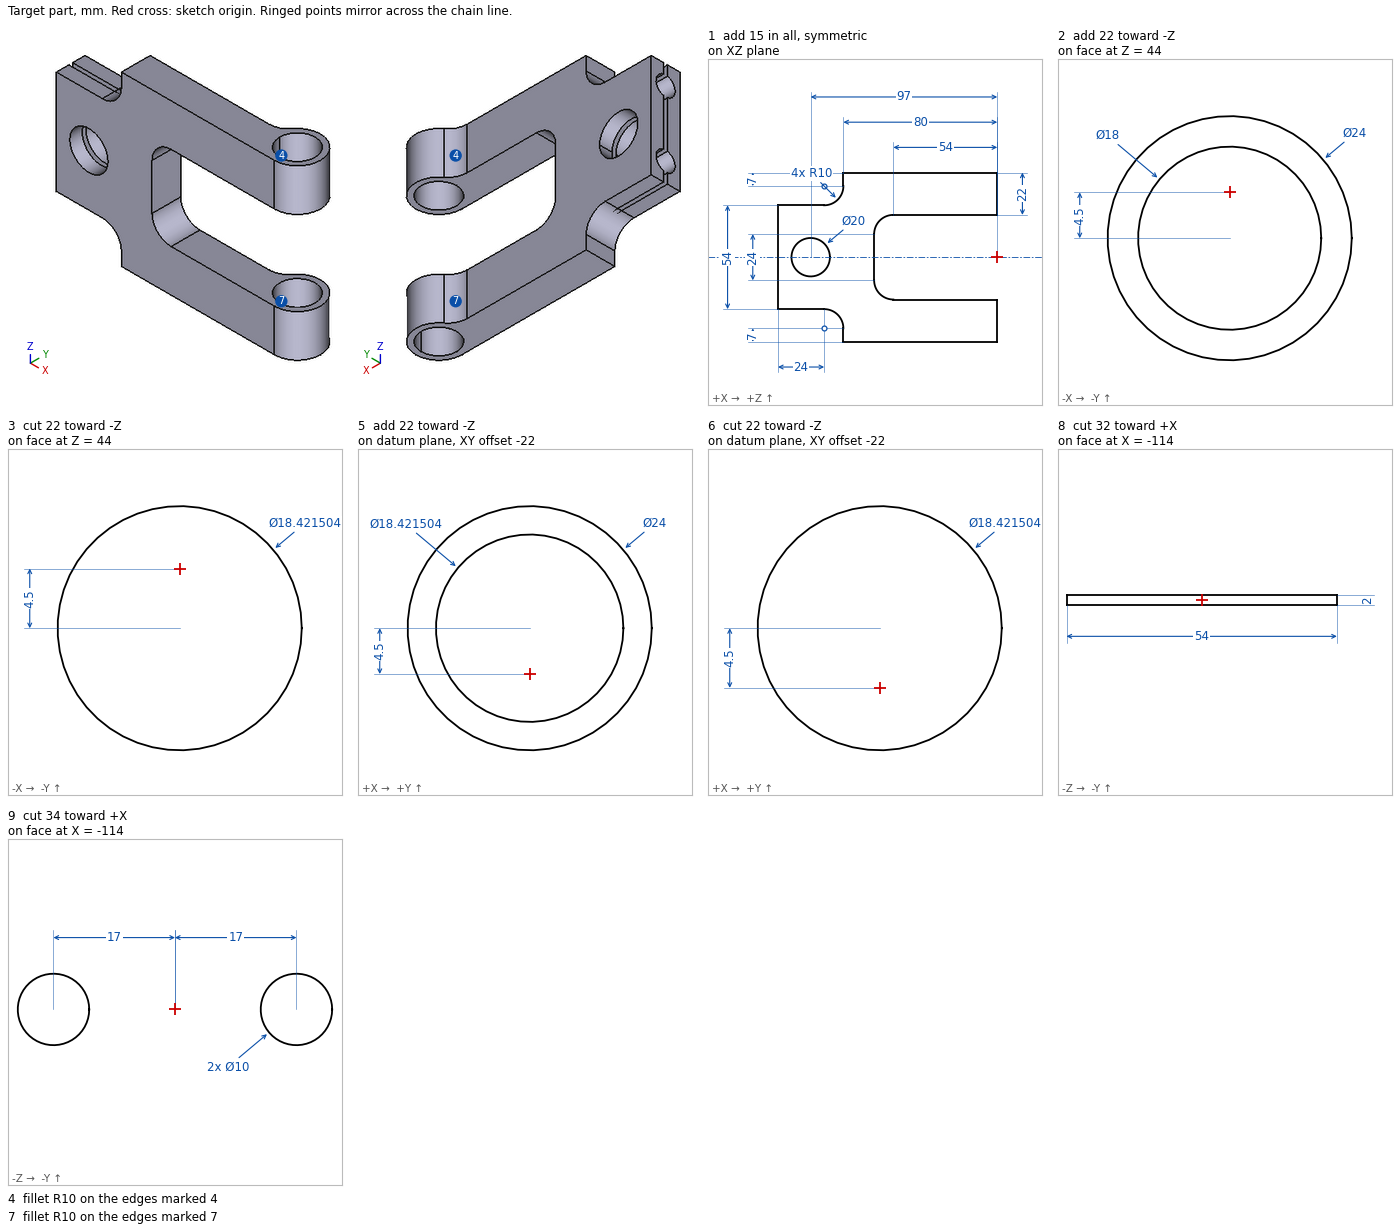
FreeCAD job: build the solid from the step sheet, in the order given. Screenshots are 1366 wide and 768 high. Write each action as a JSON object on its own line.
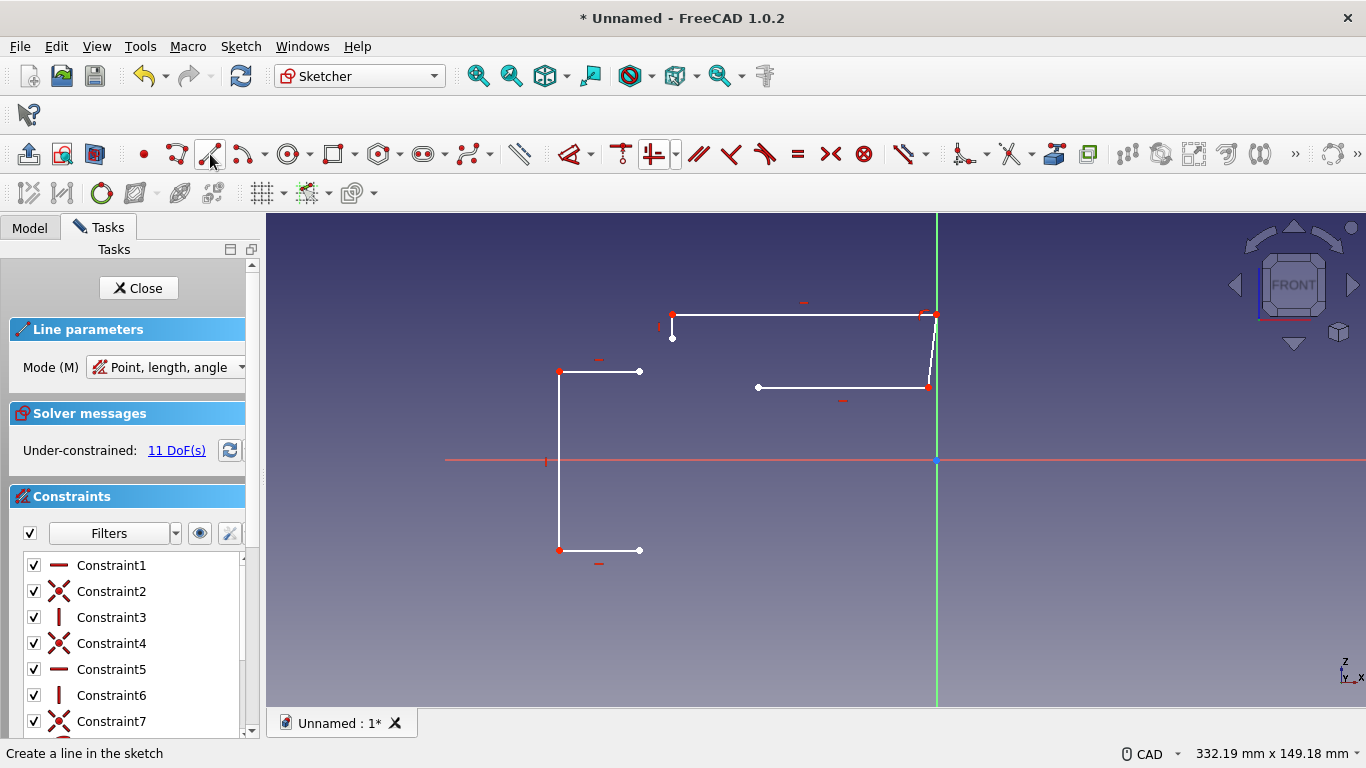
{"action": "left_click", "coordinate": [725, 420]}
{"action": "left_click", "coordinate": [725, 500]}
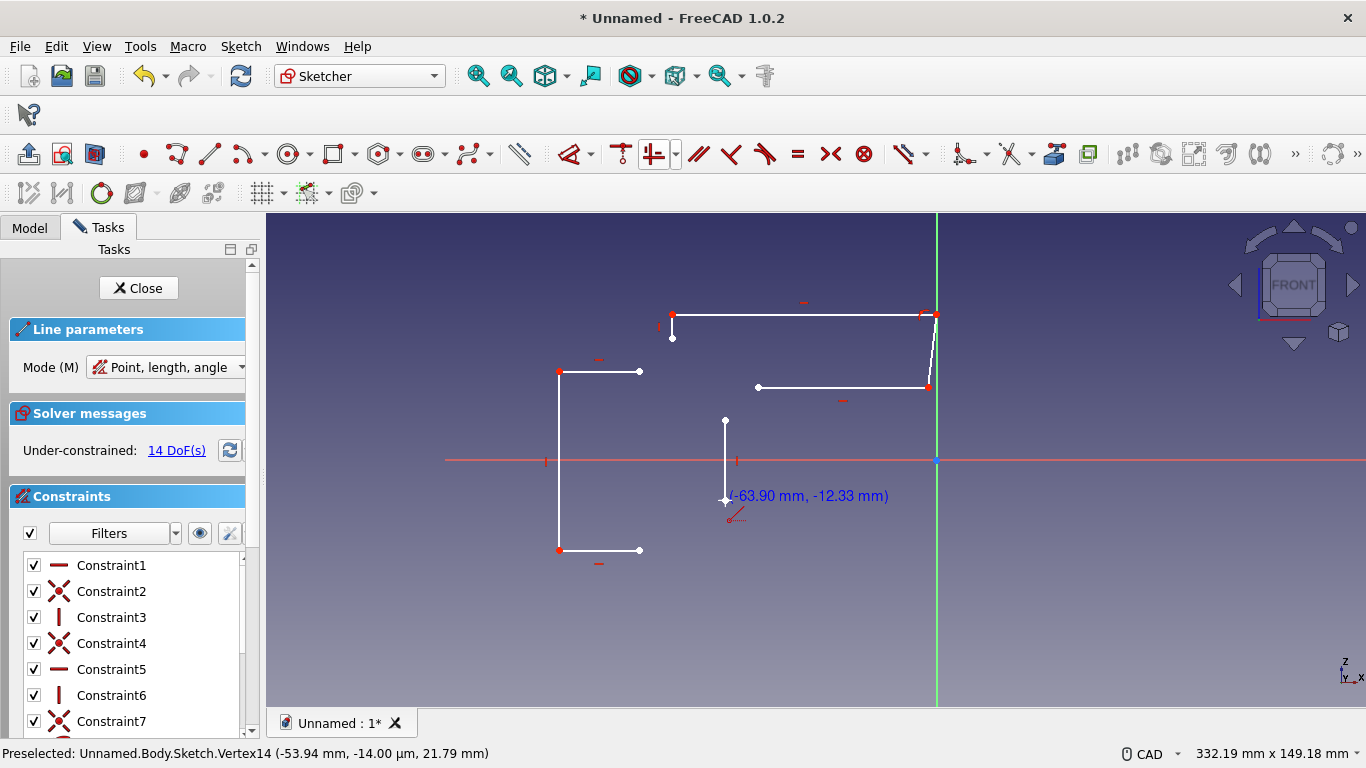
{"action": "left_click", "coordinate": [177, 154]}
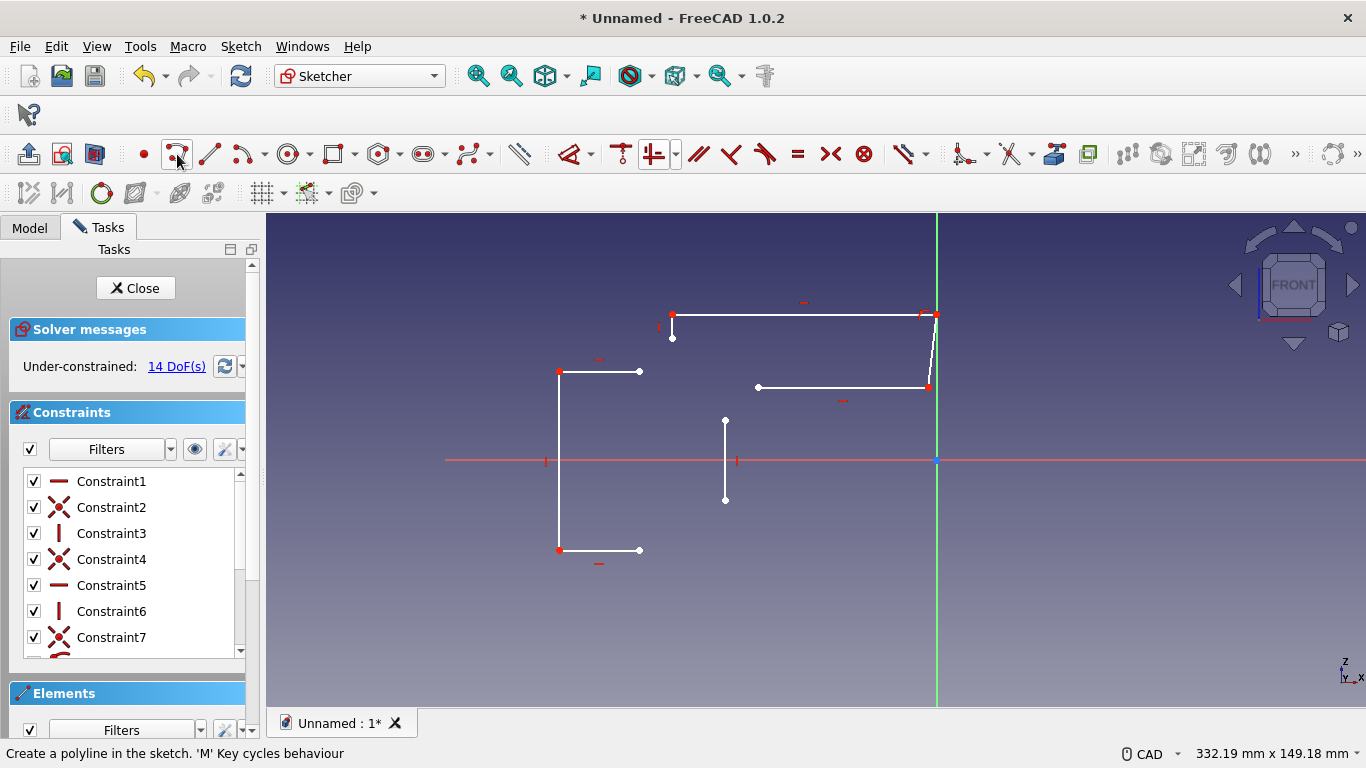
{"action": "left_click", "coordinate": [758, 533]}
{"action": "left_click", "coordinate": [937, 533]}
{"action": "left_click", "coordinate": [928, 606]}
{"action": "left_click", "coordinate": [672, 606]}
{"action": "left_click", "coordinate": [672, 583]}
{"action": "right_click", "coordinate": [672, 583]}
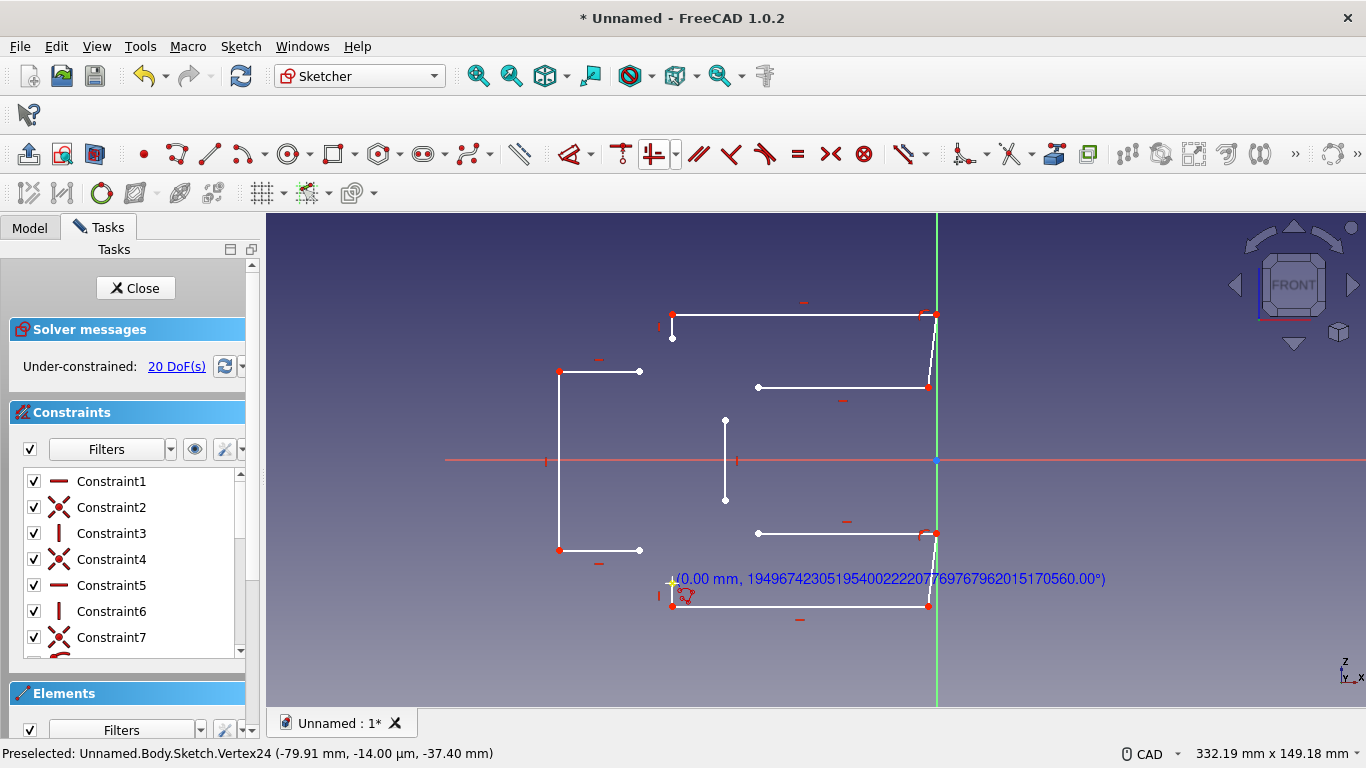
{"action": "left_click", "coordinate": [264, 154]}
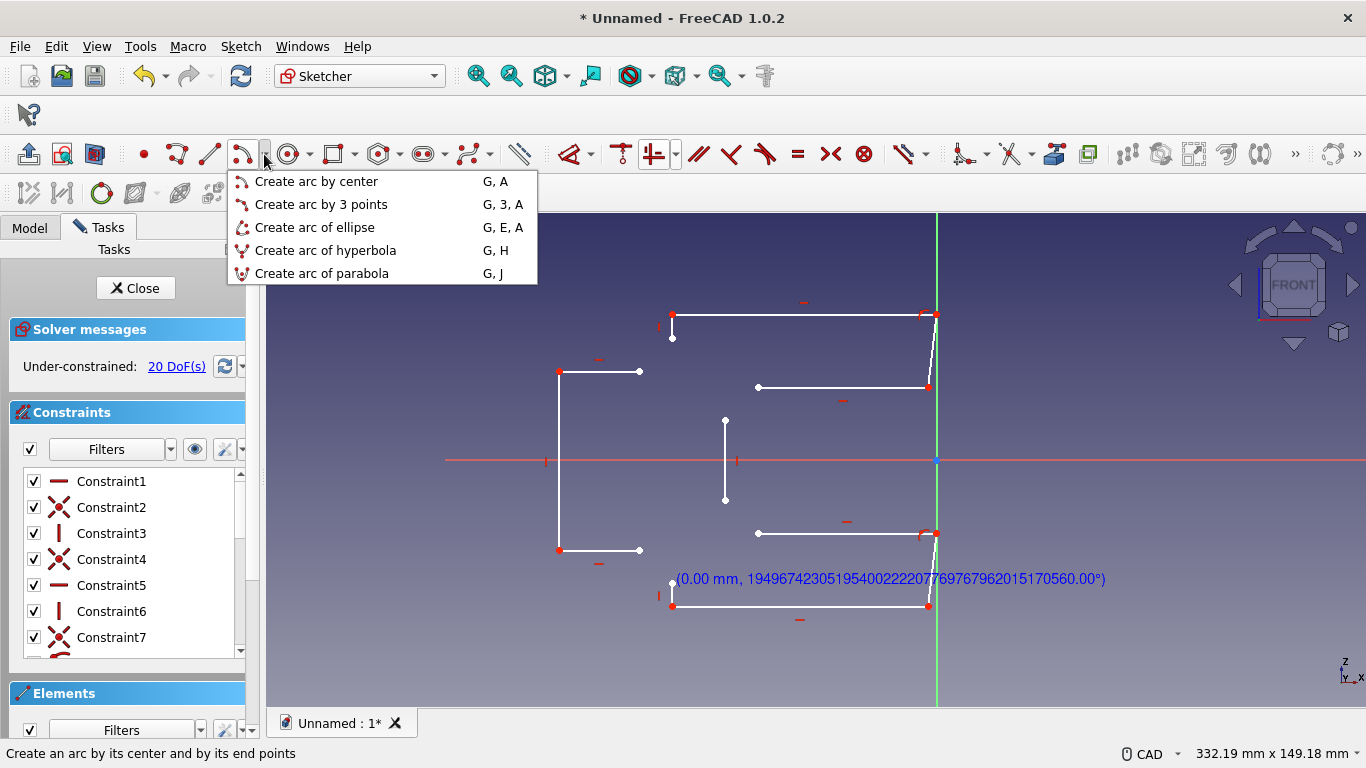
{"action": "left_click", "coordinate": [382, 204]}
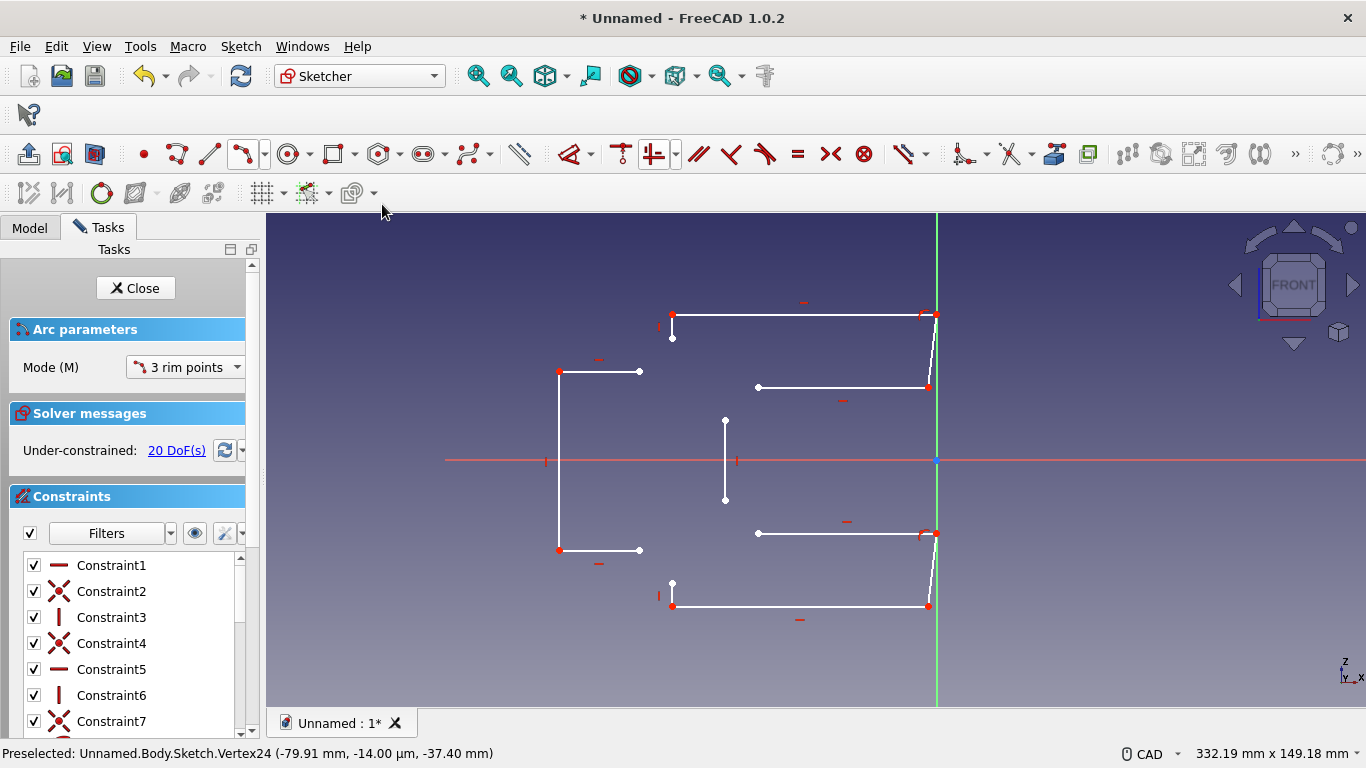
{"action": "left_click", "coordinate": [639, 372]}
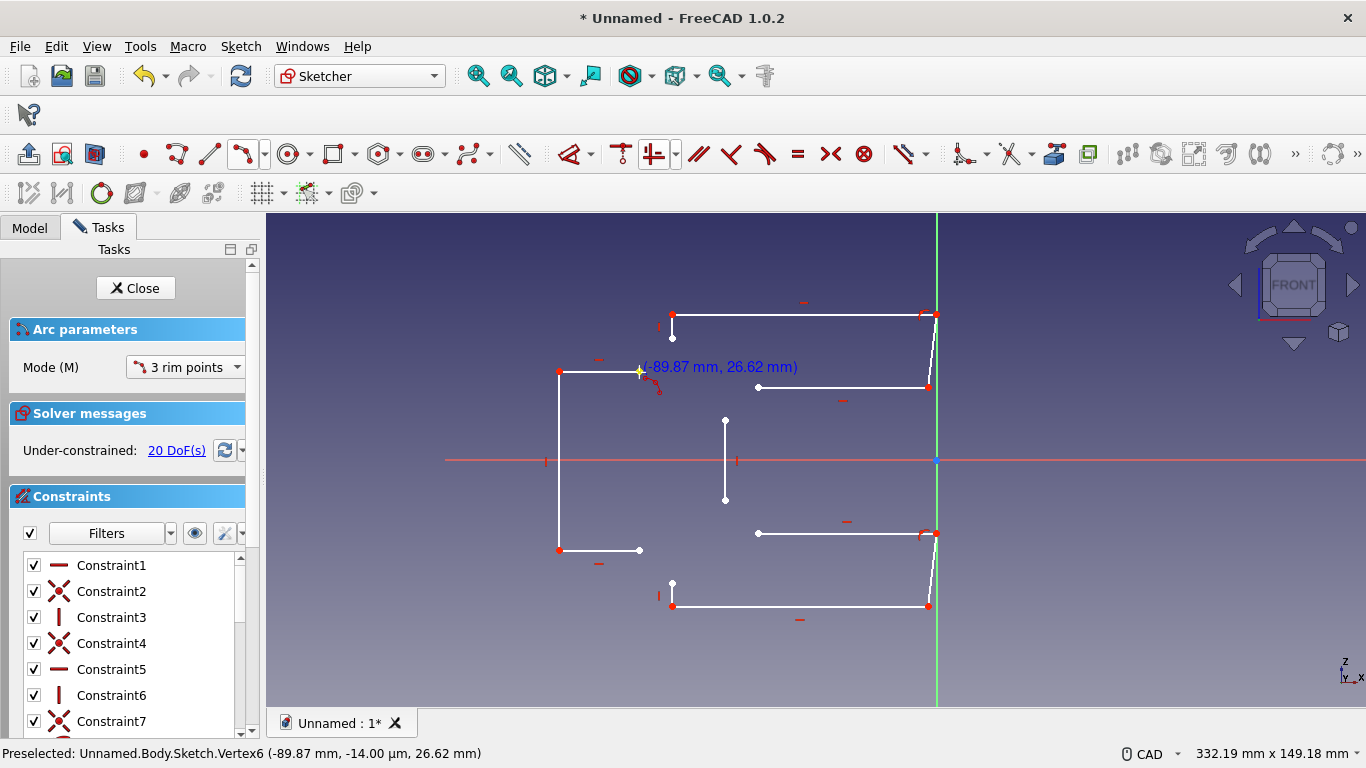
{"action": "scroll", "coordinate": [672, 338], "scroll_direction": "up", "scroll_amount": 2}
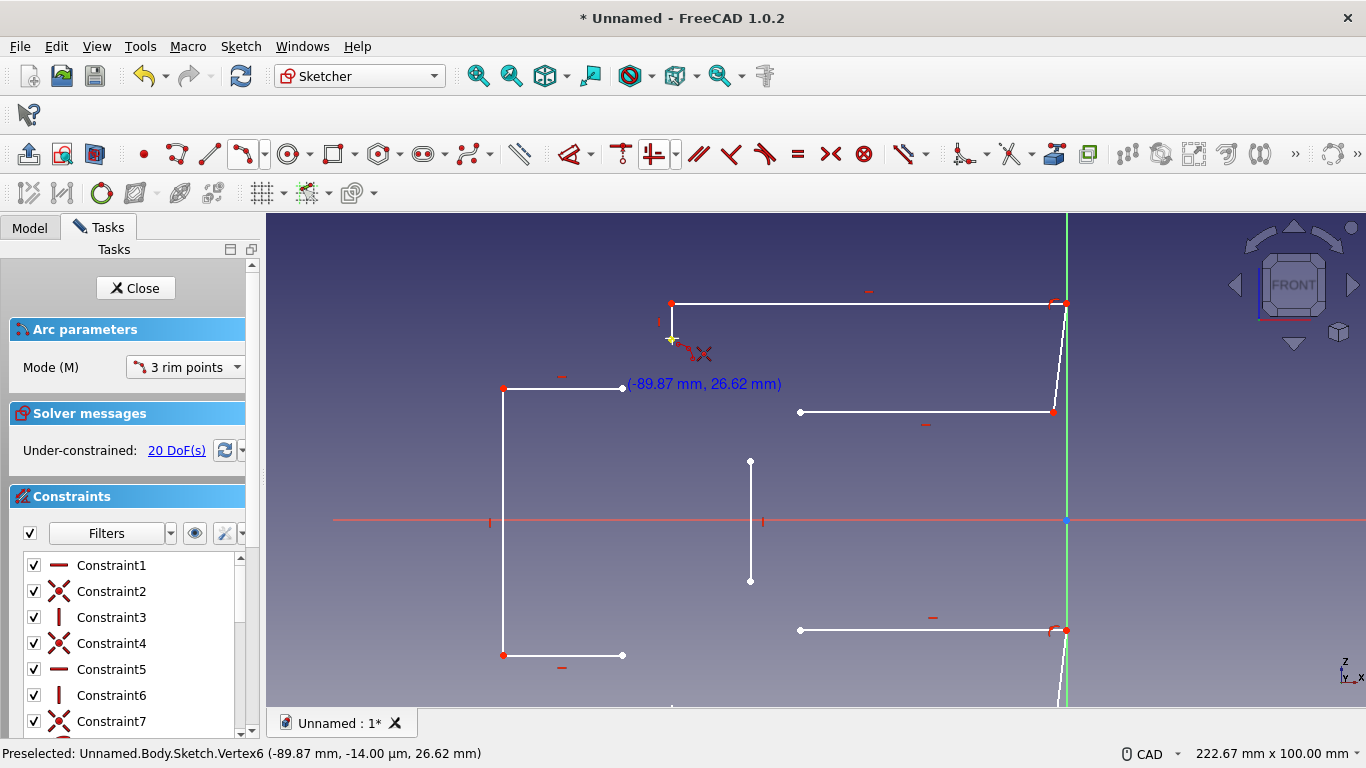
{"action": "left_click", "coordinate": [672, 339]}
{"action": "left_click", "coordinate": [657, 372]}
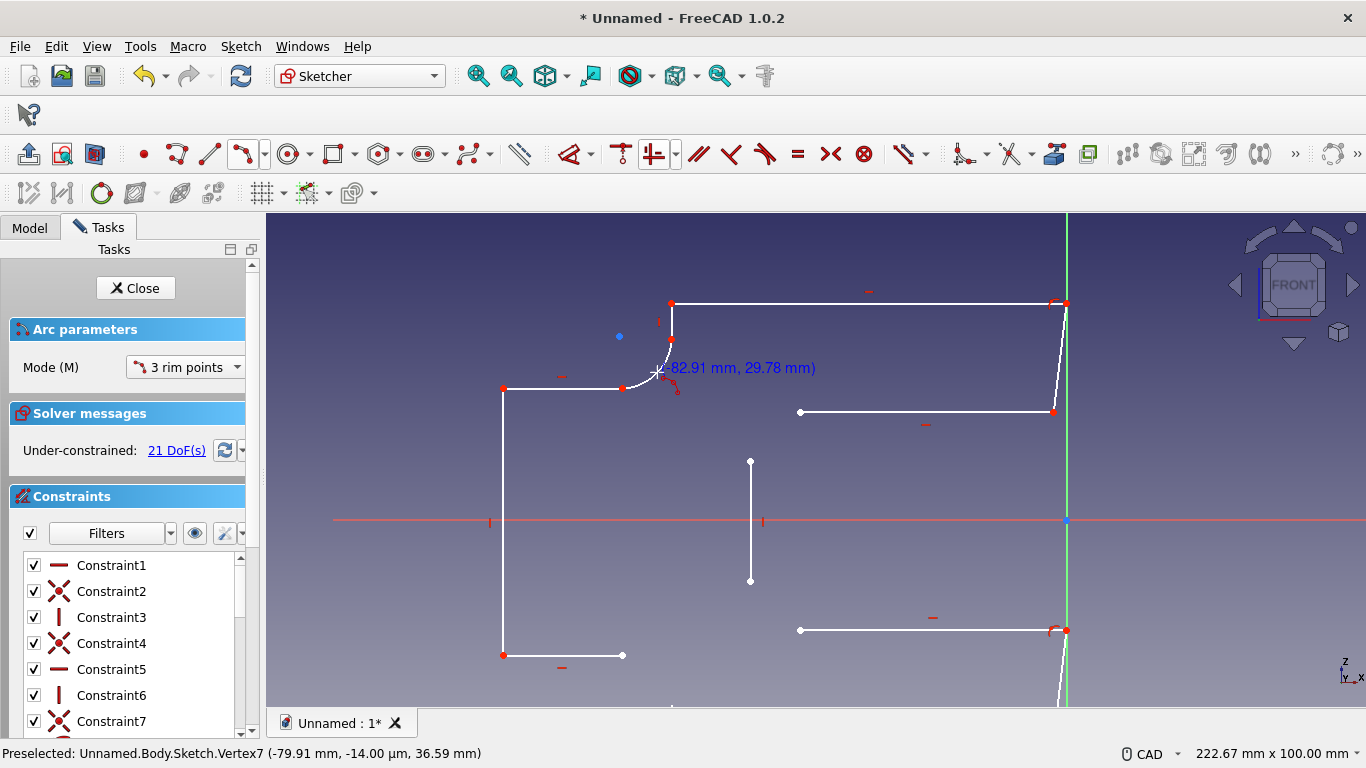
{"action": "left_click", "coordinate": [800, 412]}
{"action": "left_click", "coordinate": [751, 462]}
{"action": "left_click", "coordinate": [765, 426]}